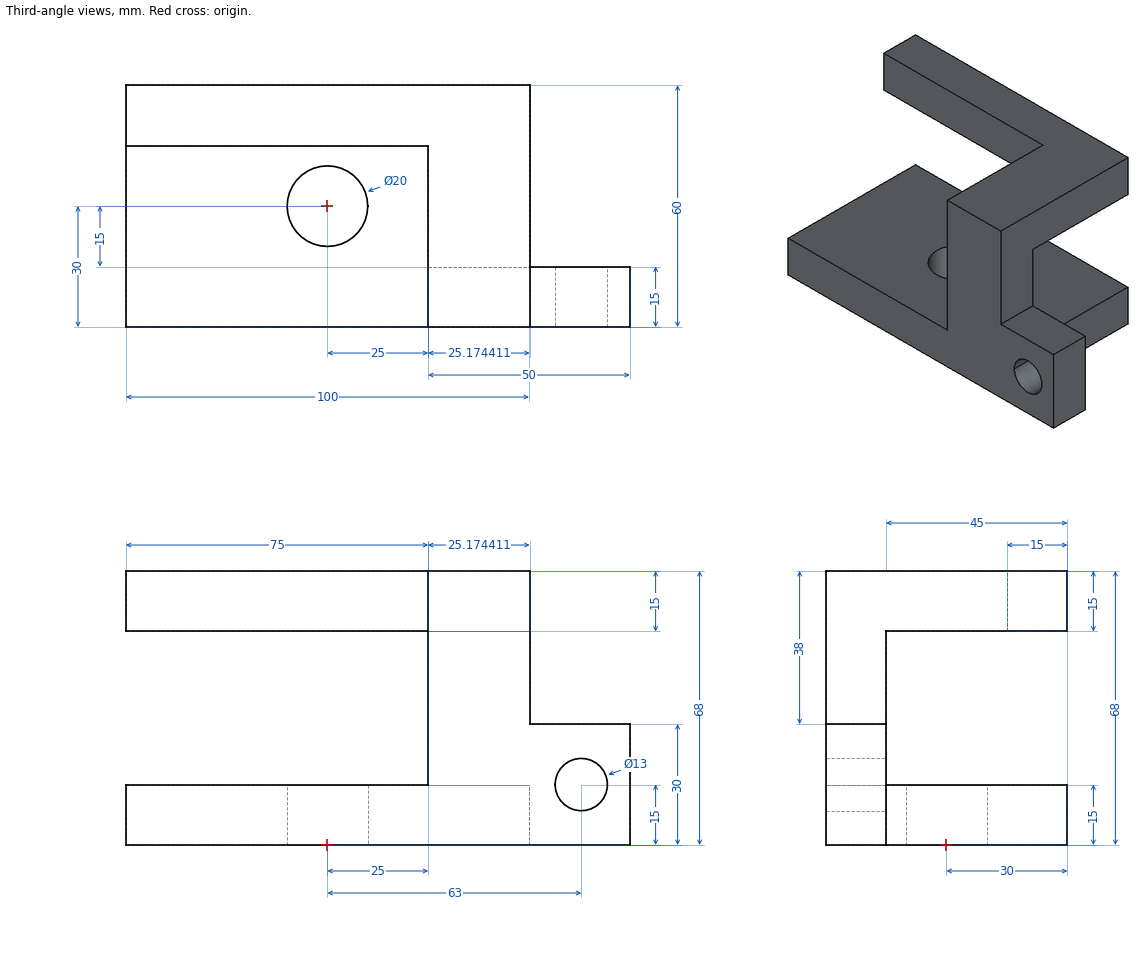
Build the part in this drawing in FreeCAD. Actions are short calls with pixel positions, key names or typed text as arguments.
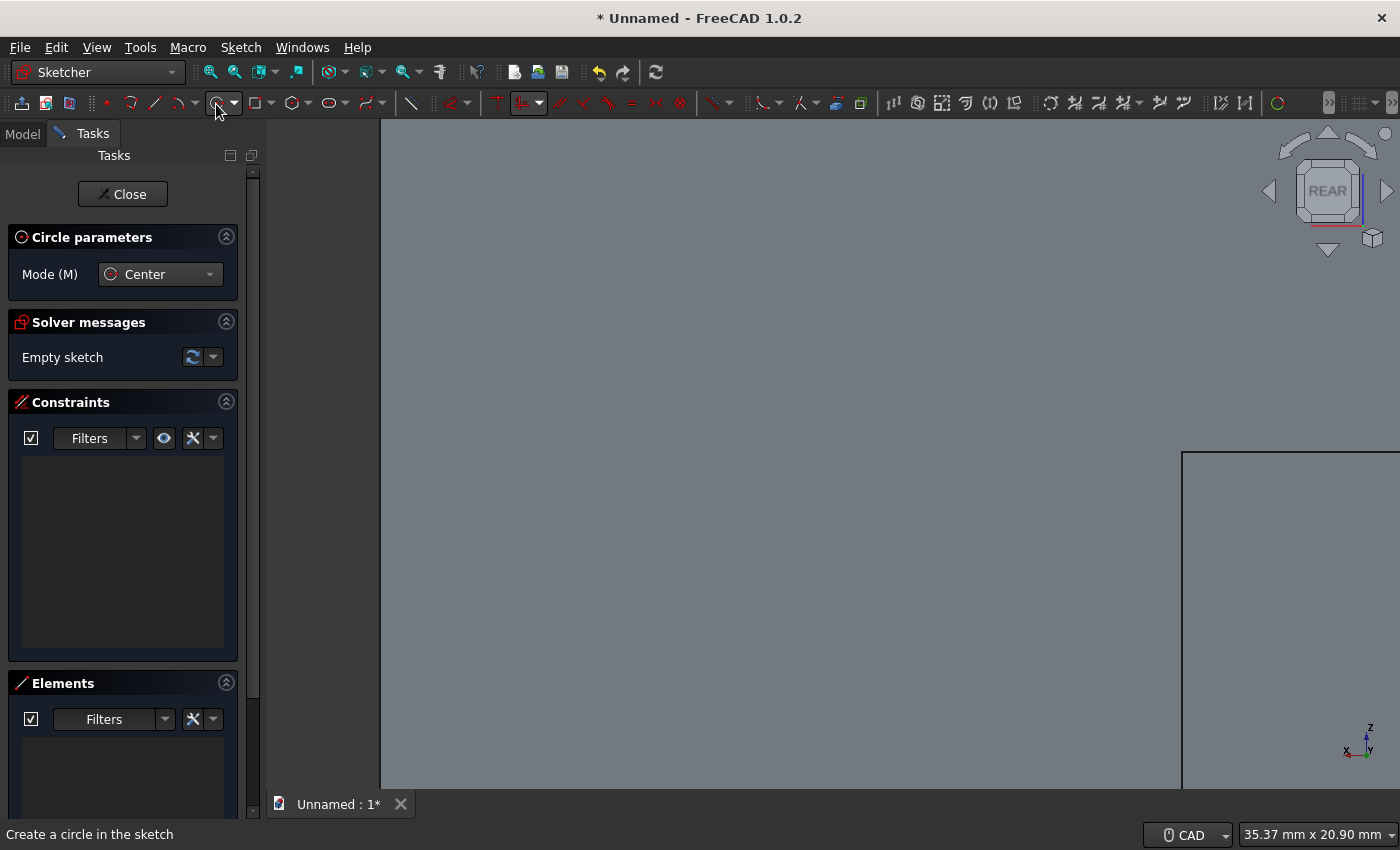
click(765, 452)
move(912, 305)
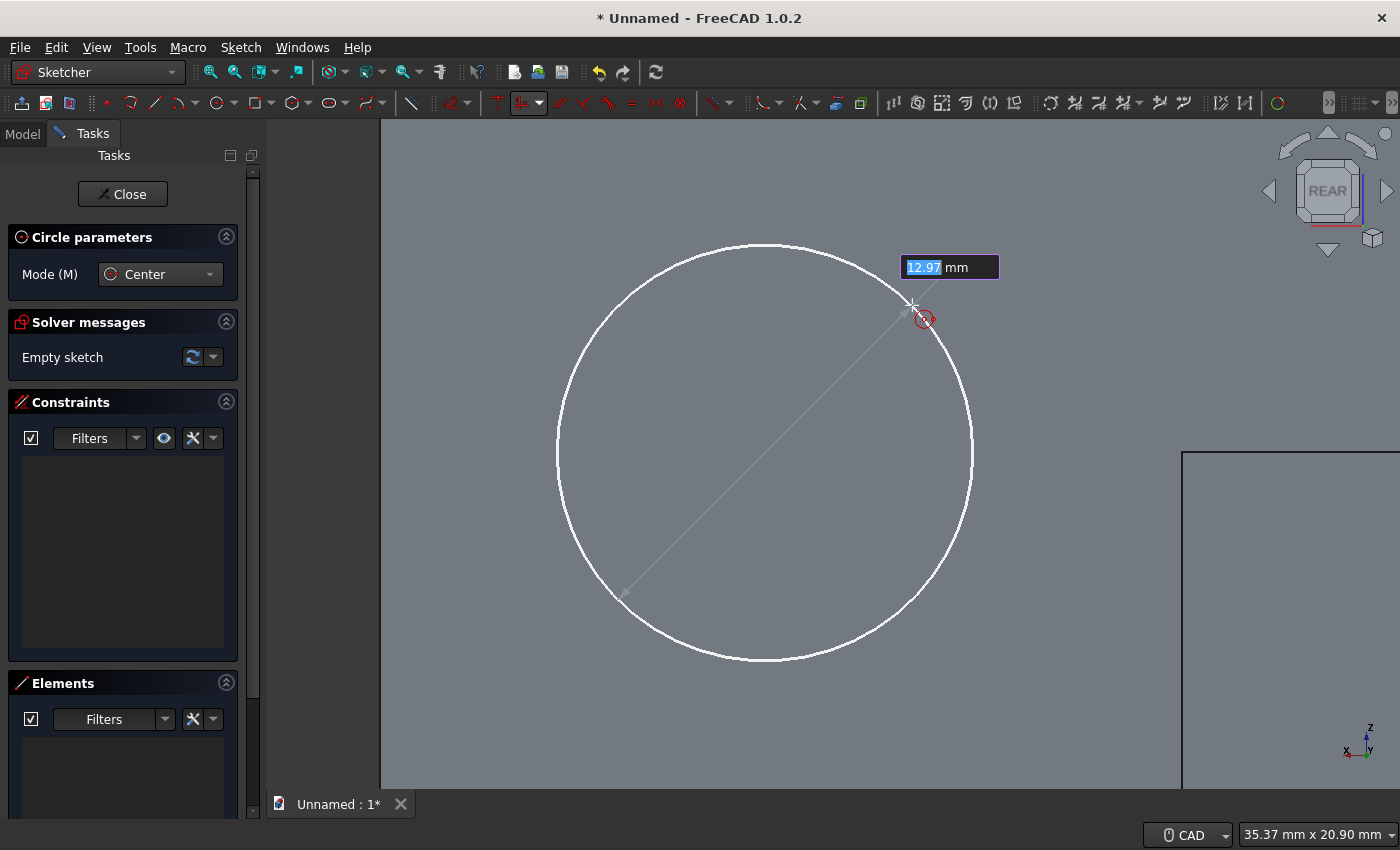
text(13)
key(Return)
key(Escape)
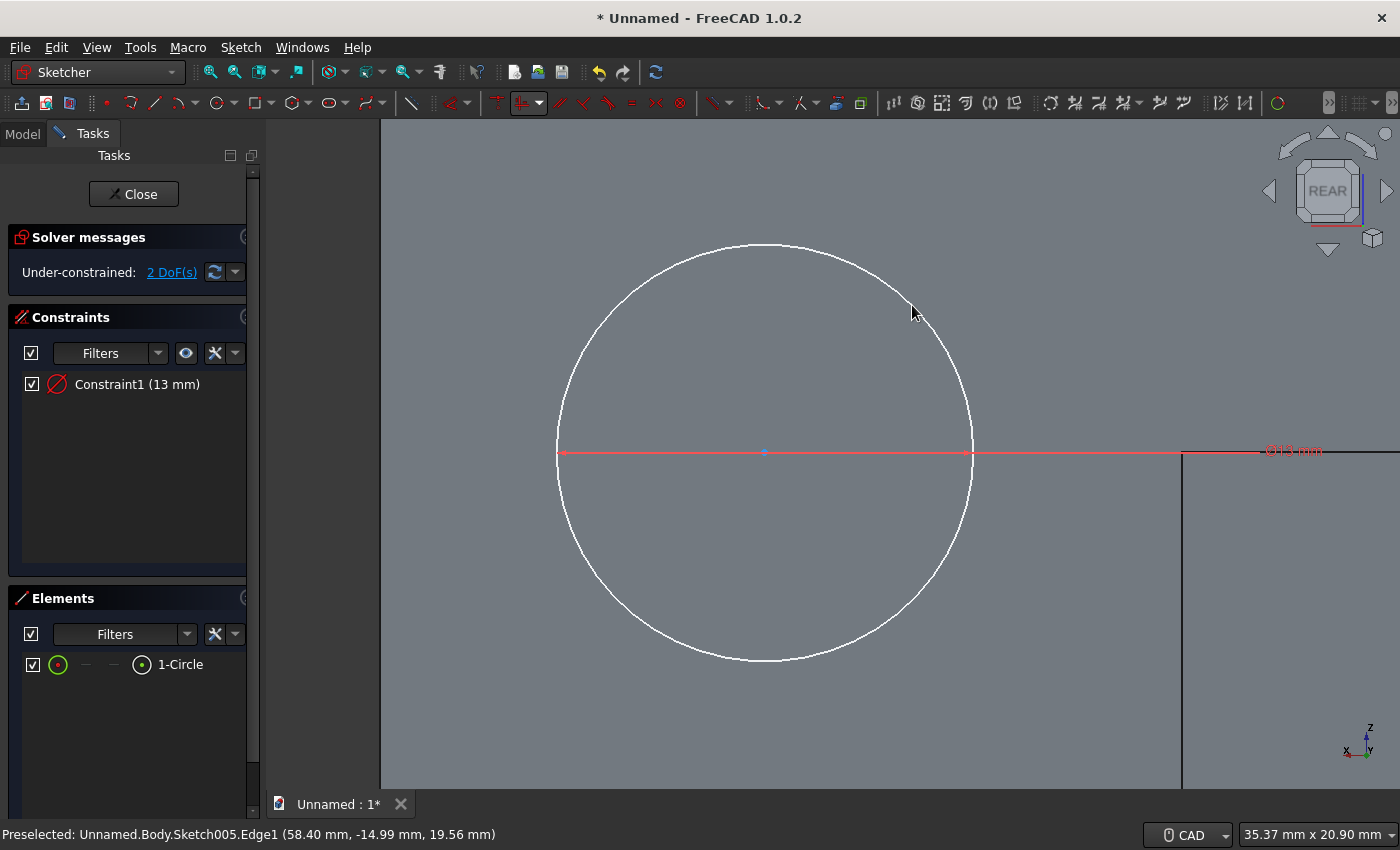
click(450, 104)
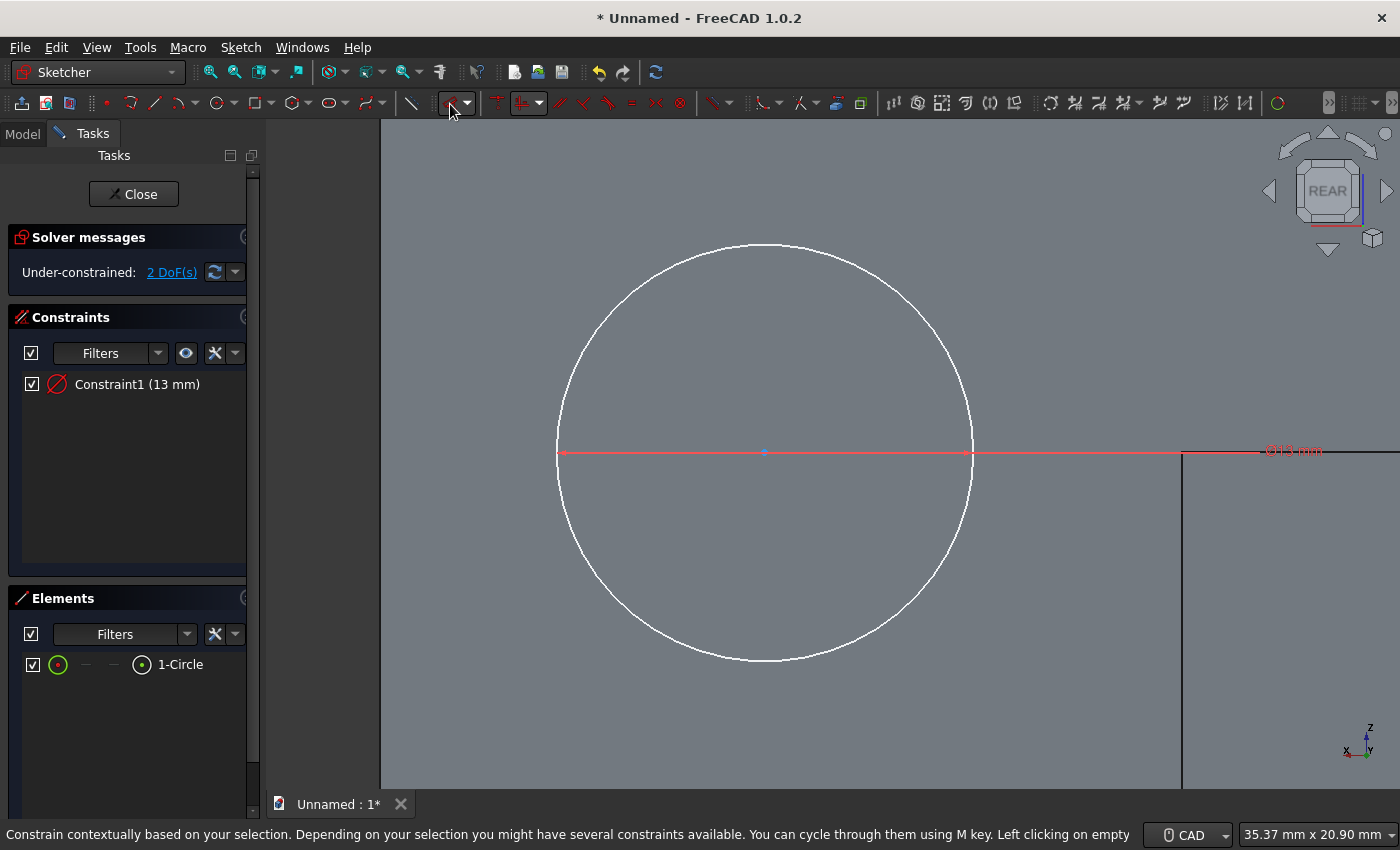
click(765, 453)
click(1000, 419)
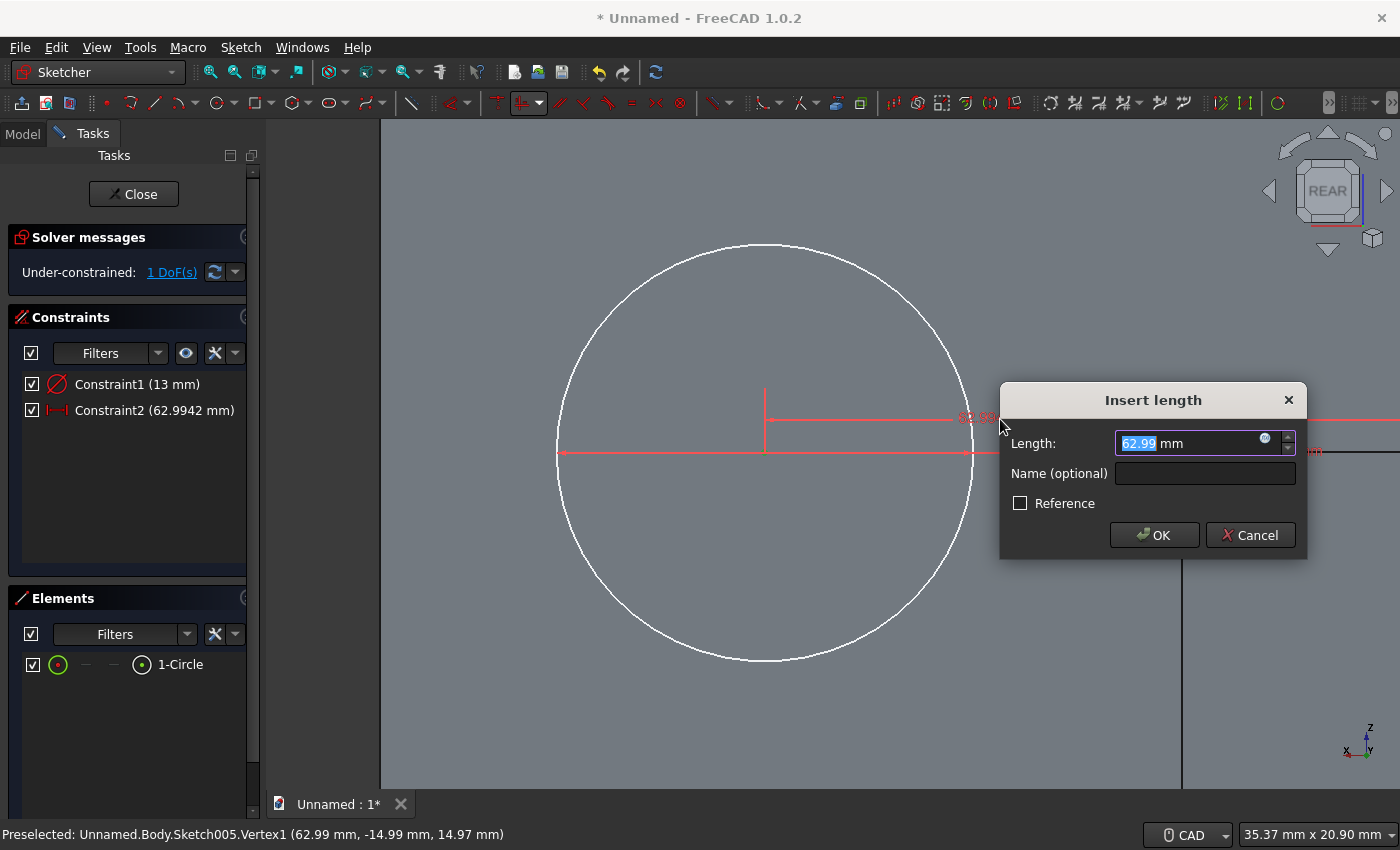
text(63)
key(Return)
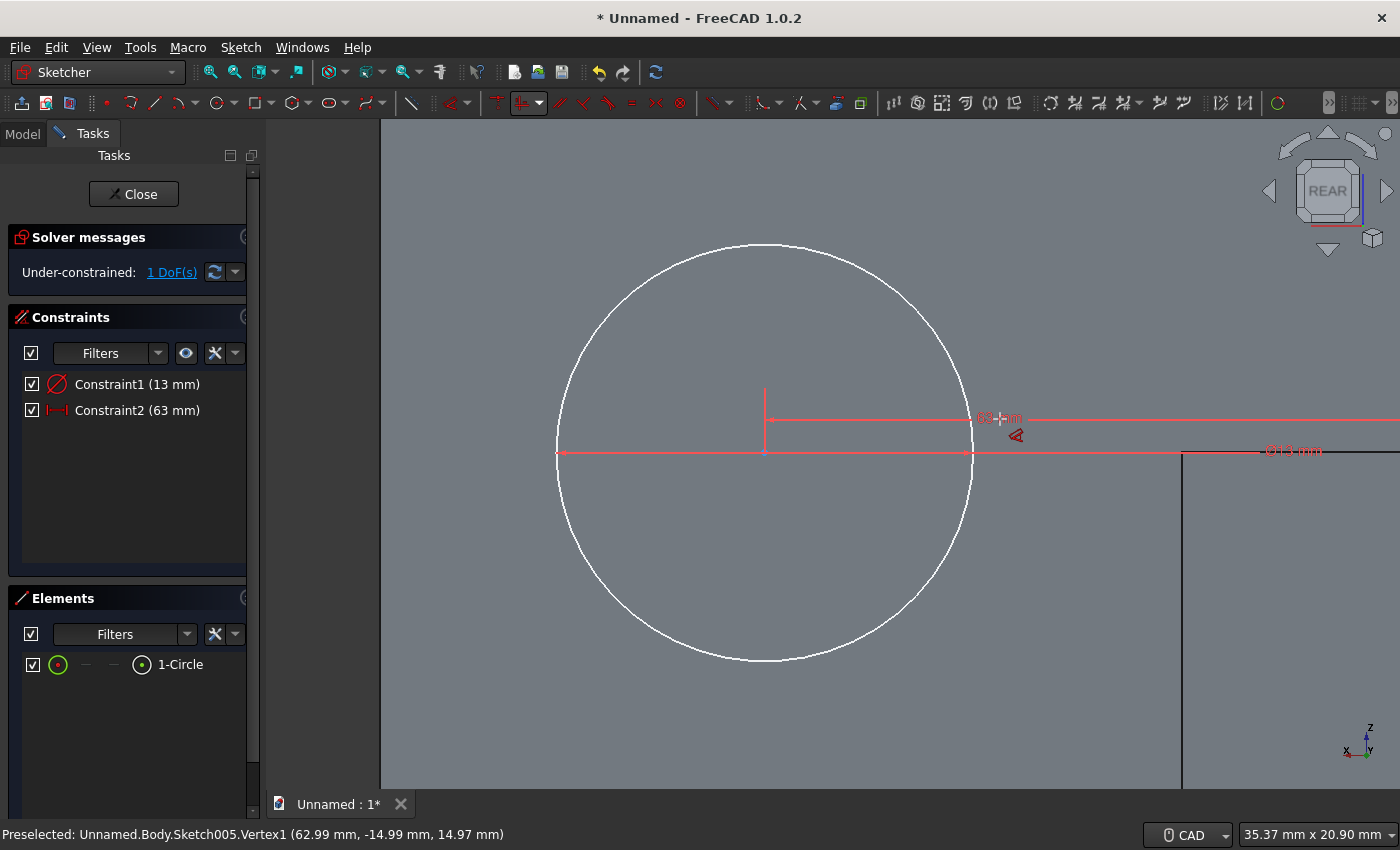
click(765, 453)
click(731, 607)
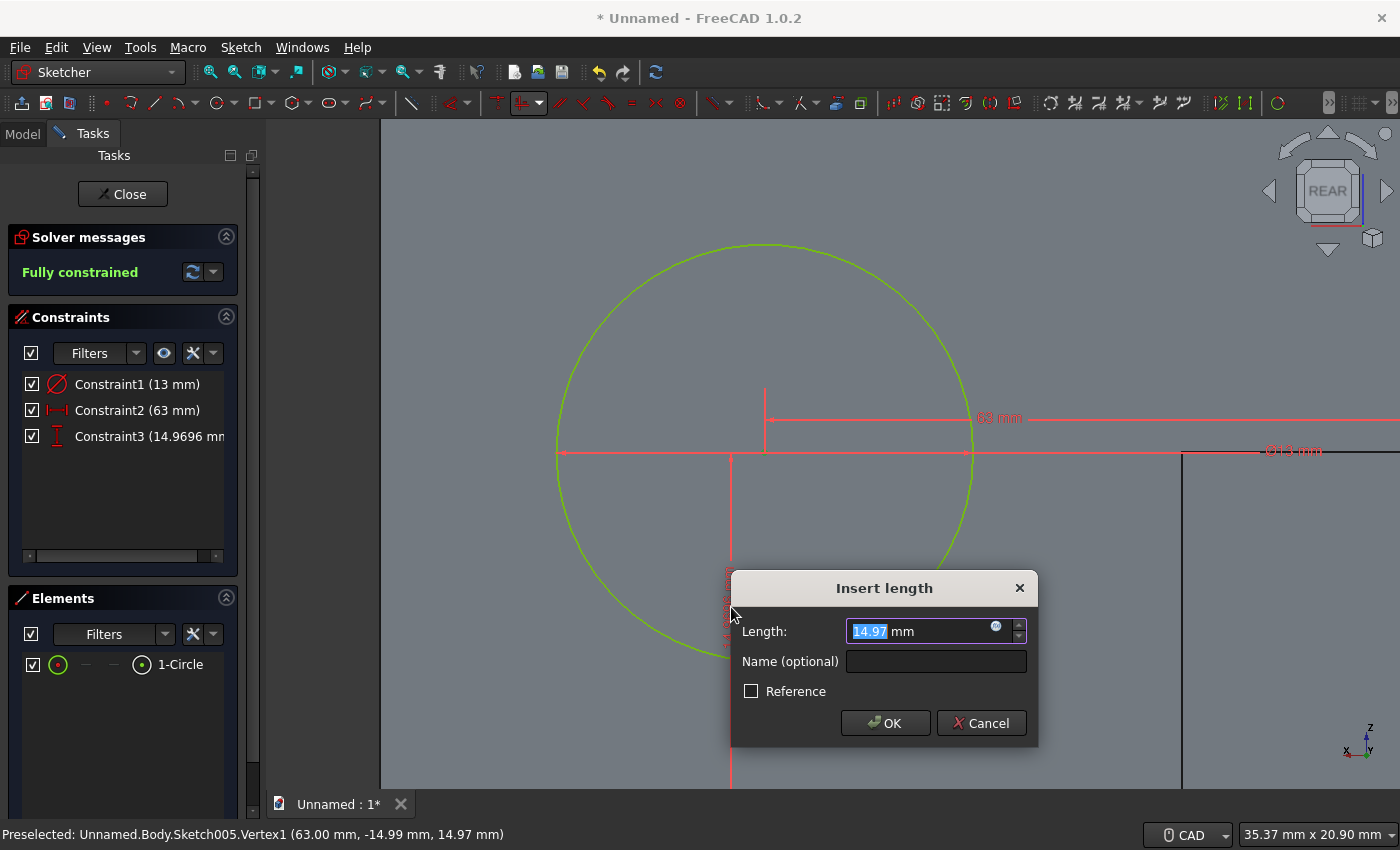
text(15)
key(Return)
key(Escape)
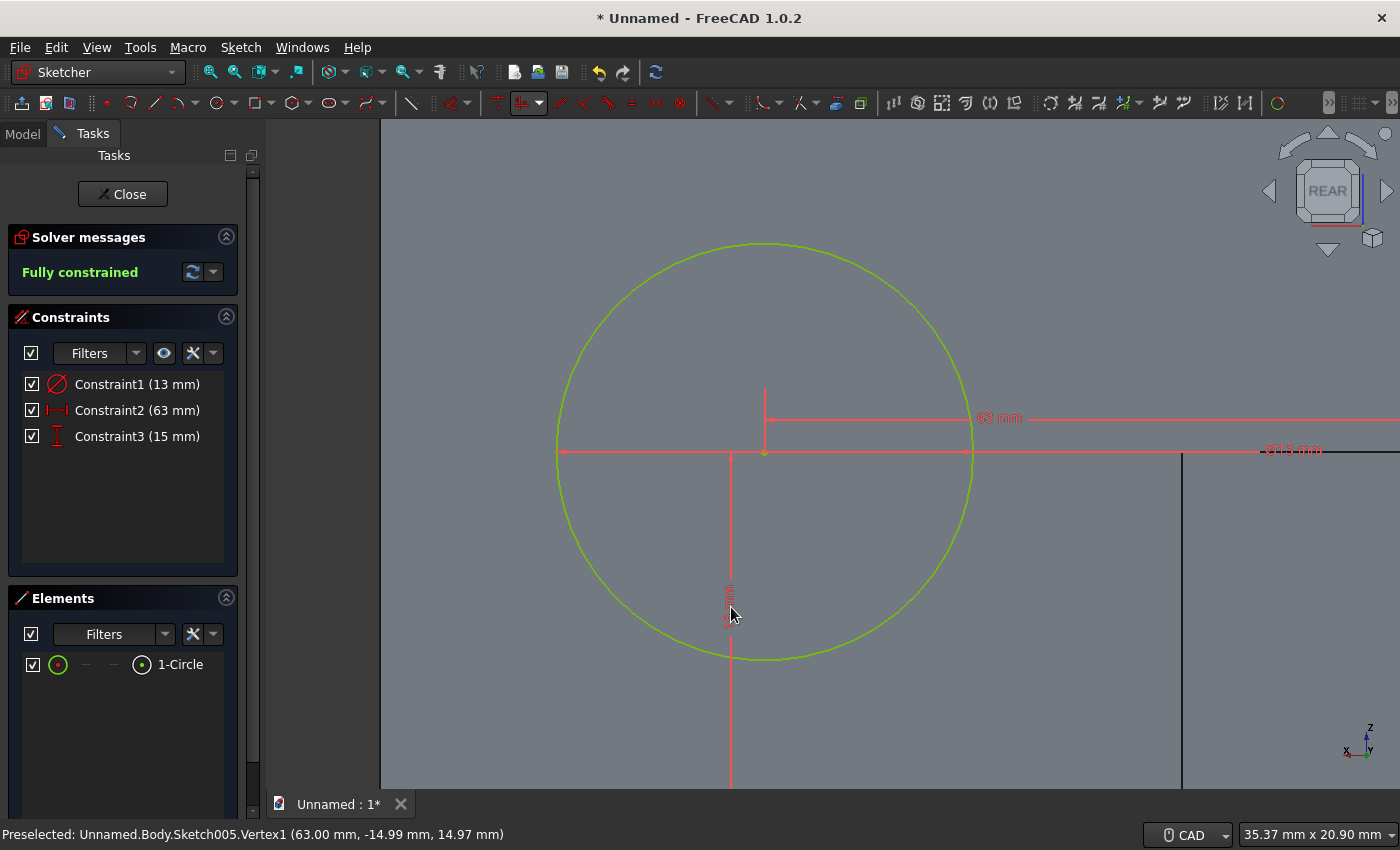
click(123, 194)